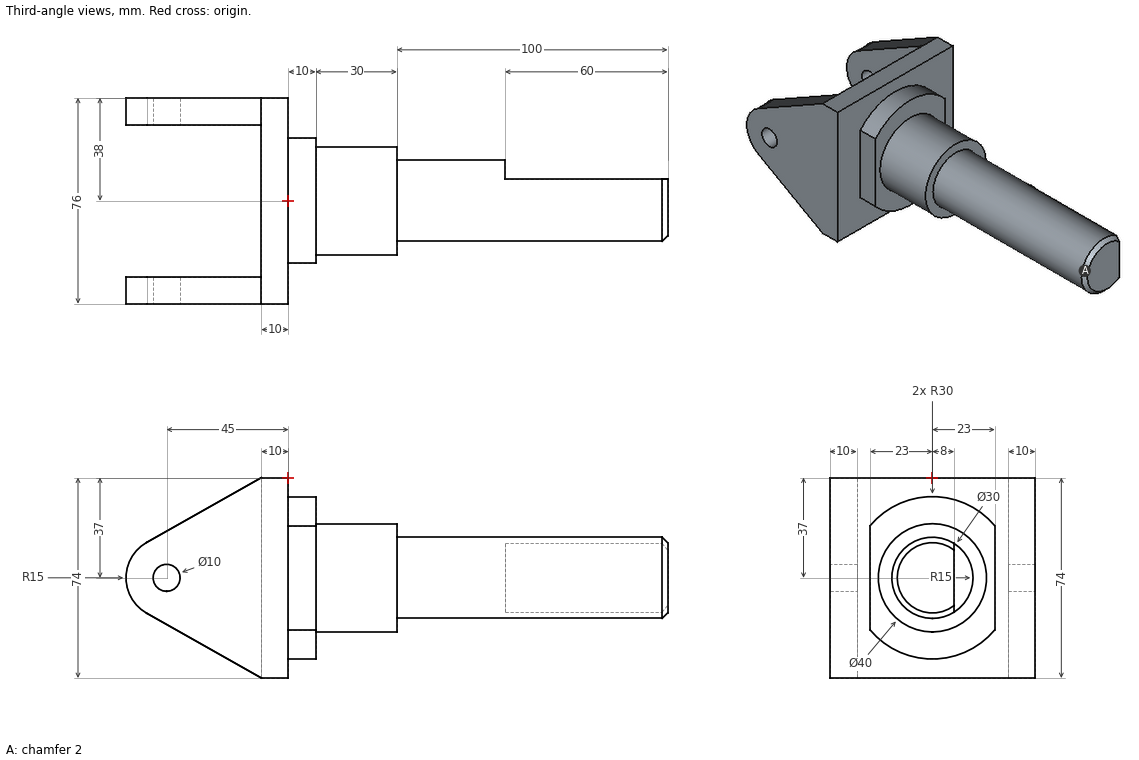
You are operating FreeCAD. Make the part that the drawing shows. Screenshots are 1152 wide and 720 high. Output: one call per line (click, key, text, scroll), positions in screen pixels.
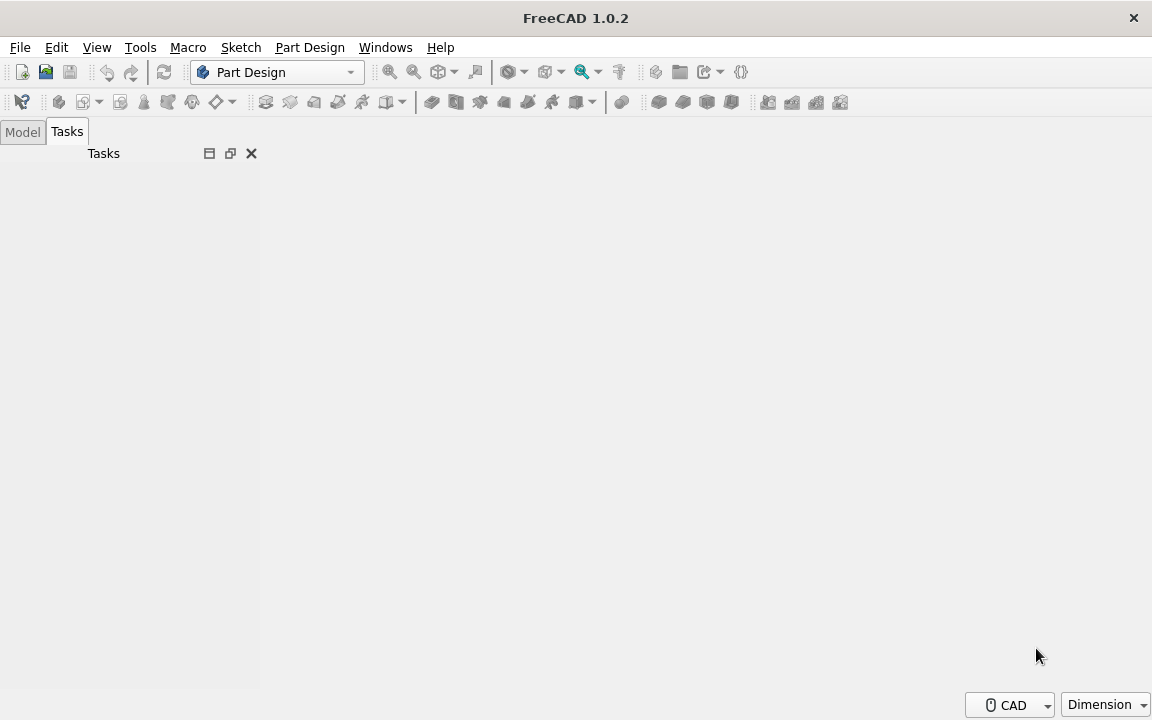
click(22, 72)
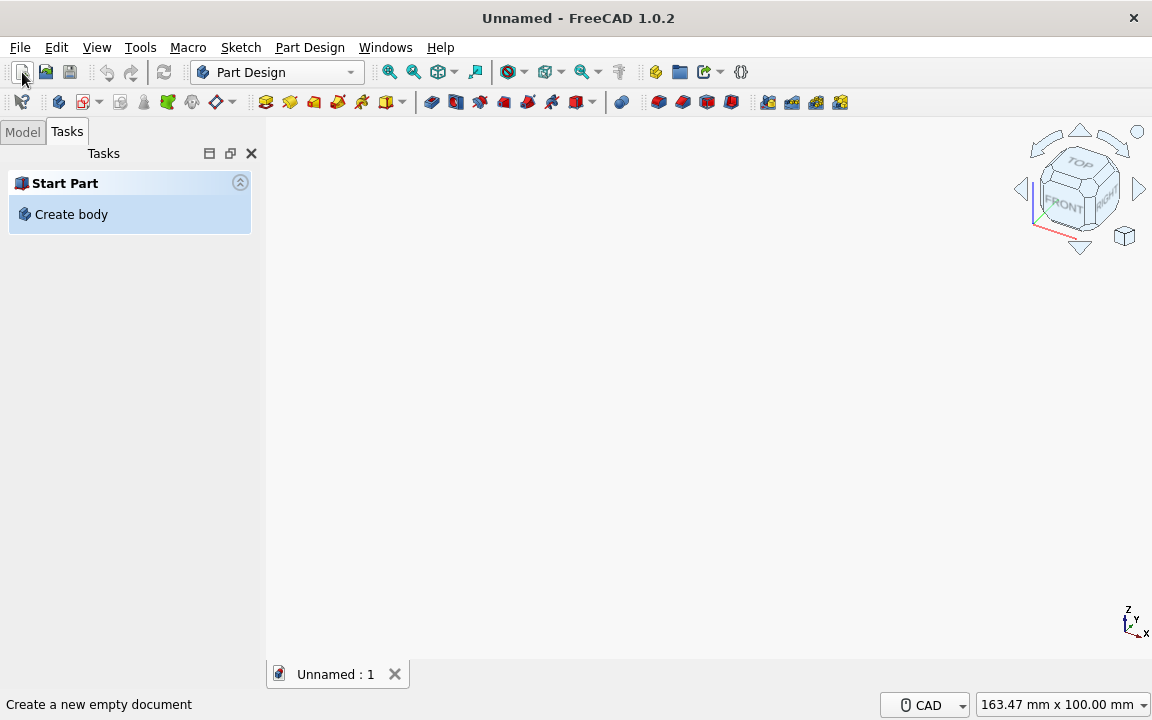
click(84, 102)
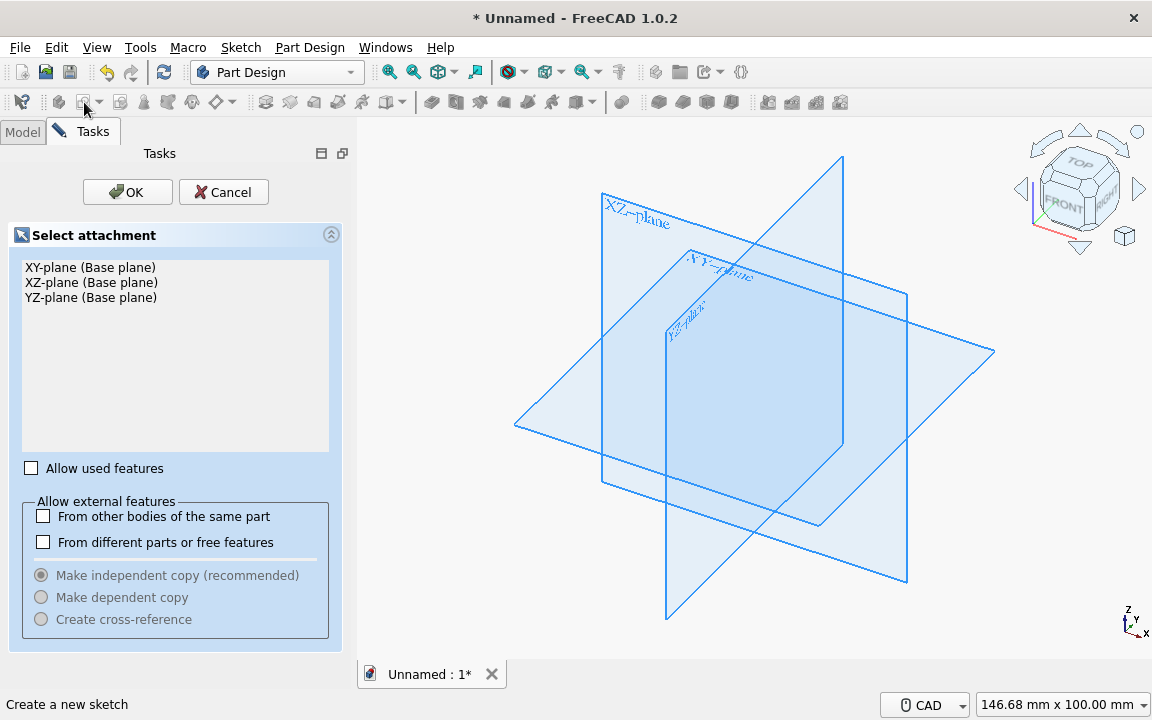
click(82, 268)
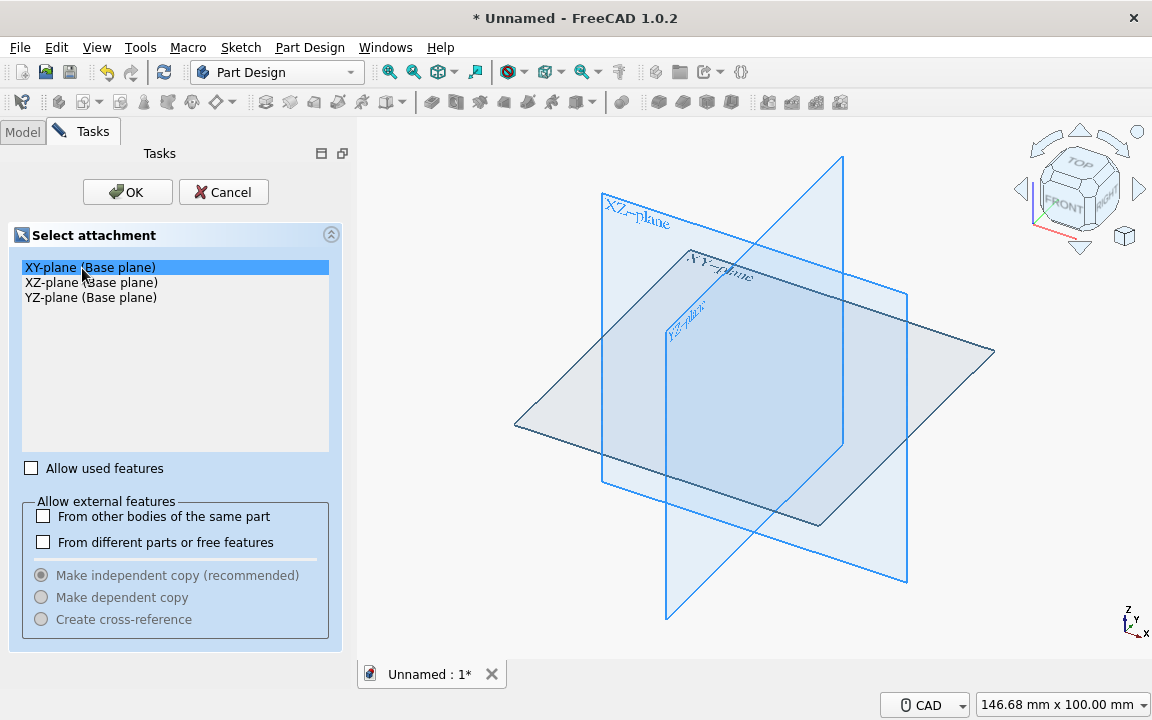
click(128, 192)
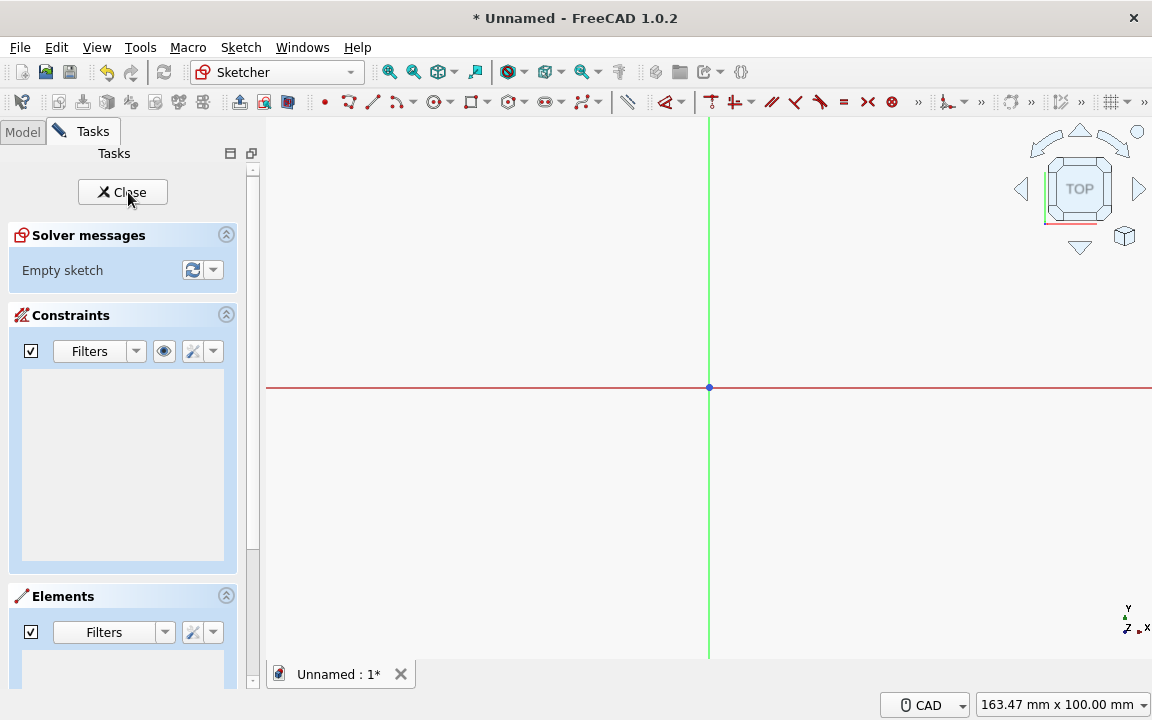
click(472, 102)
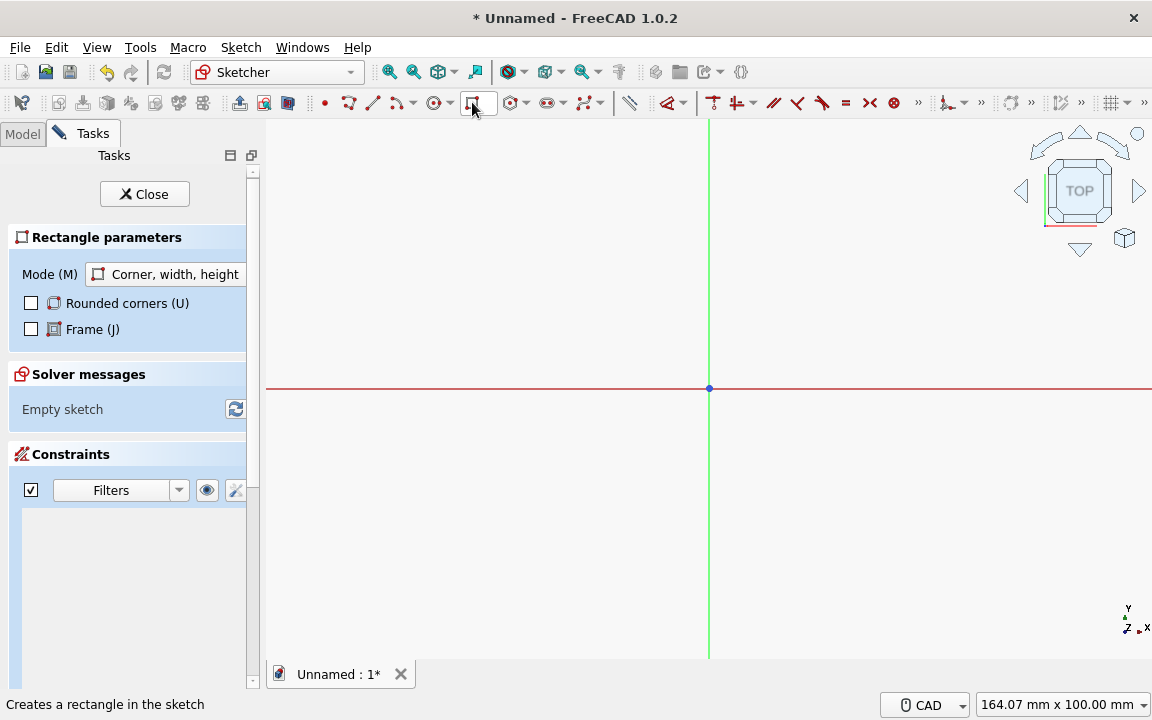
click(655, 184)
click(709, 594)
key(Escape)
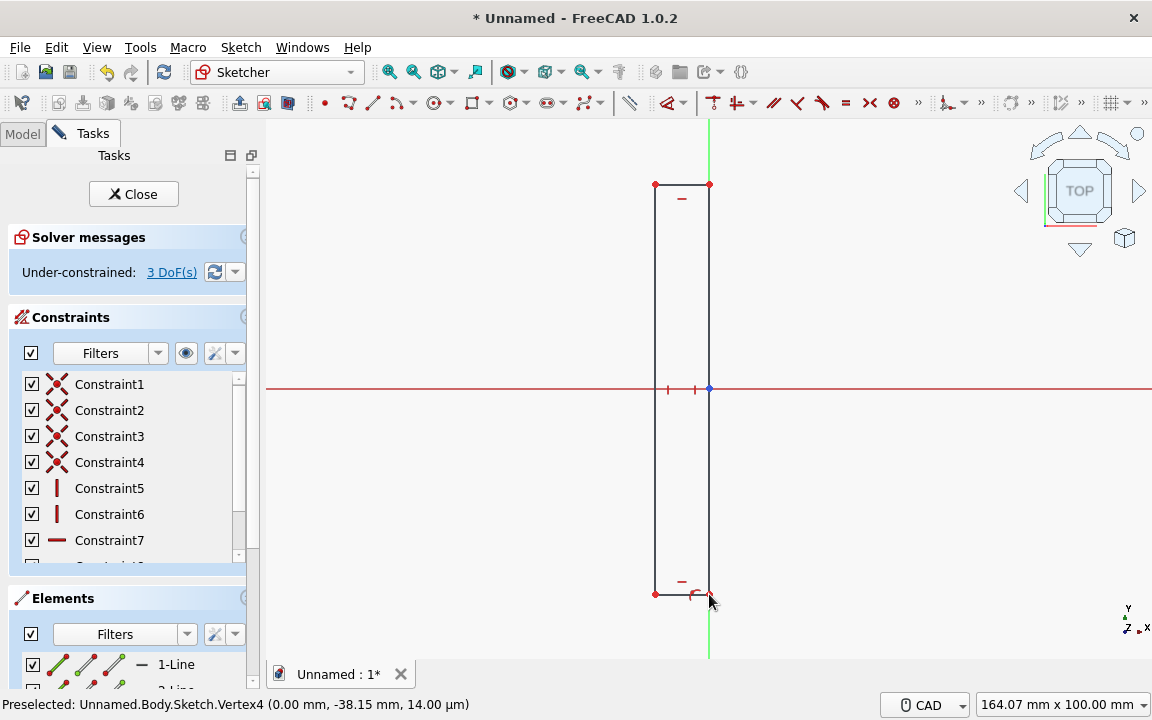
click(668, 104)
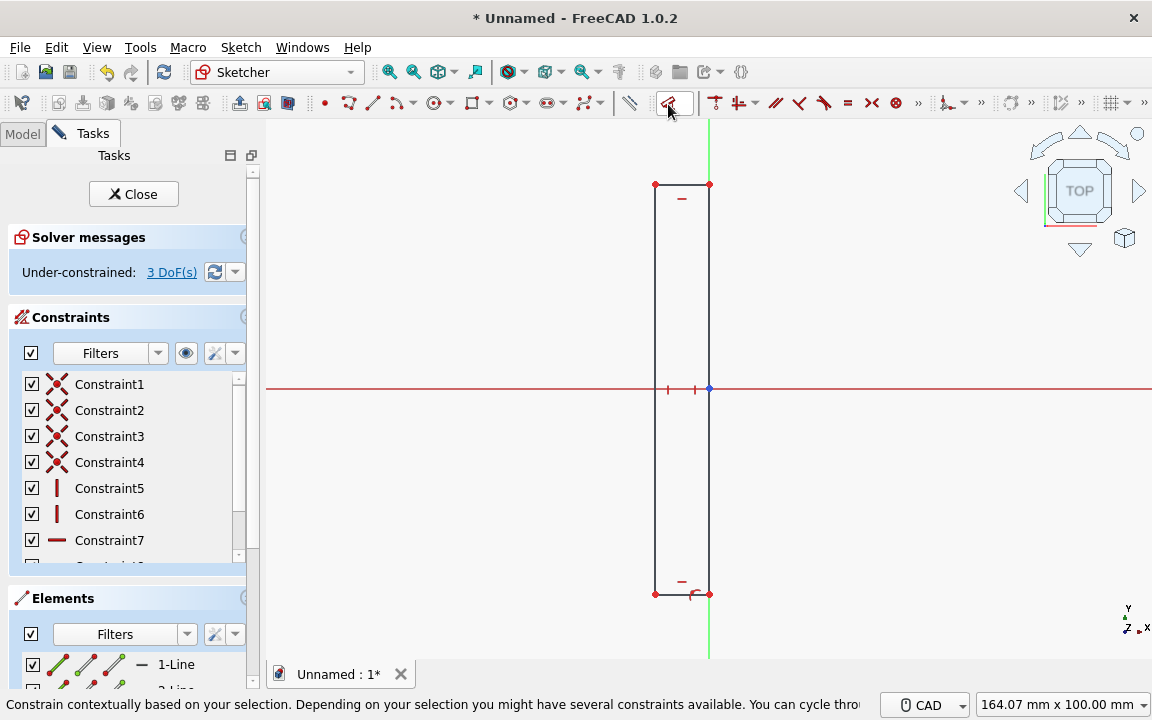
click(655, 308)
click(621, 296)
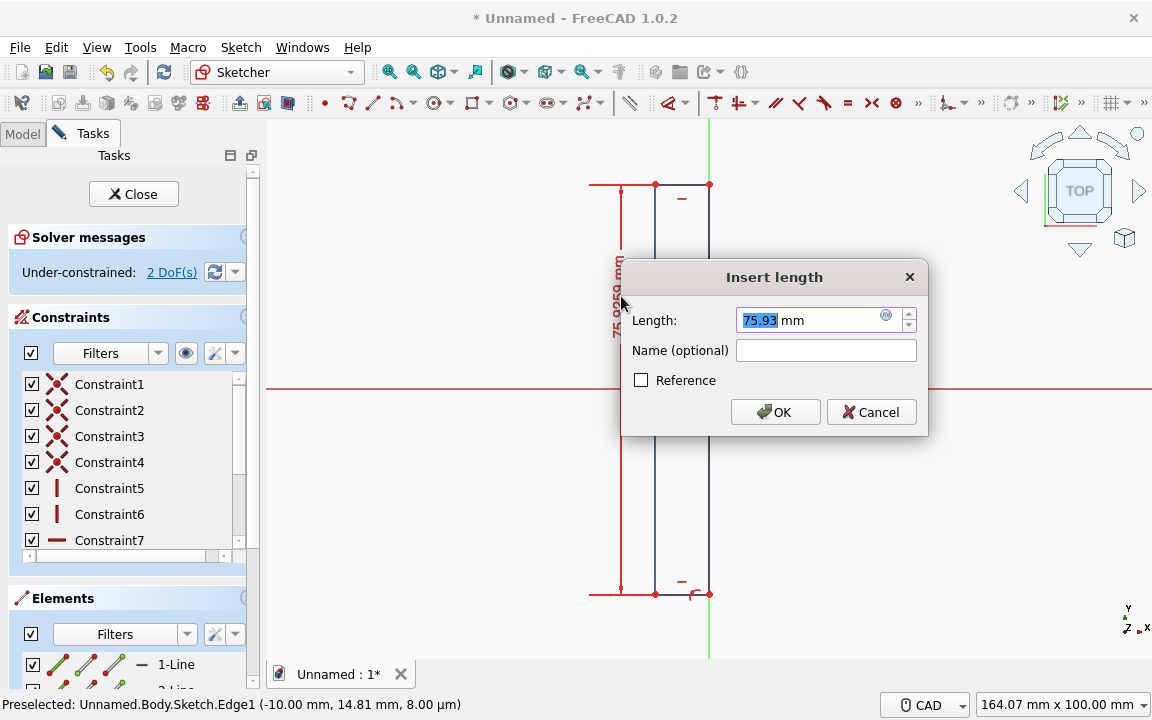
text(76)
key(Return)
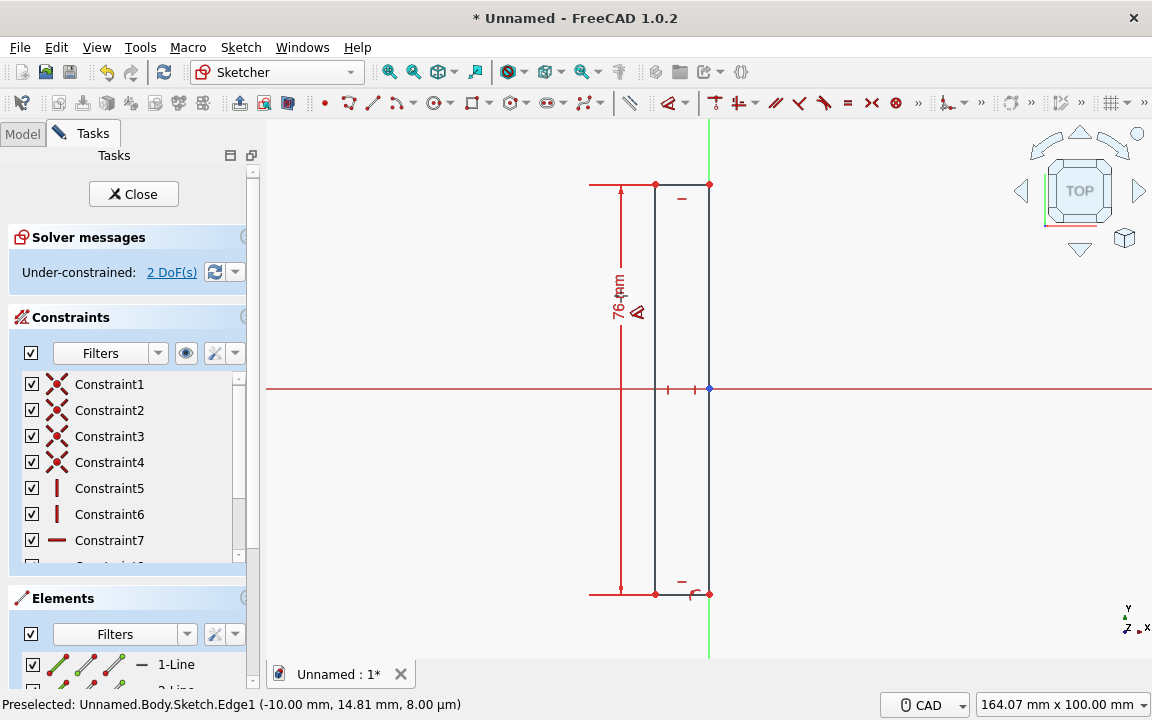
click(671, 595)
click(682, 629)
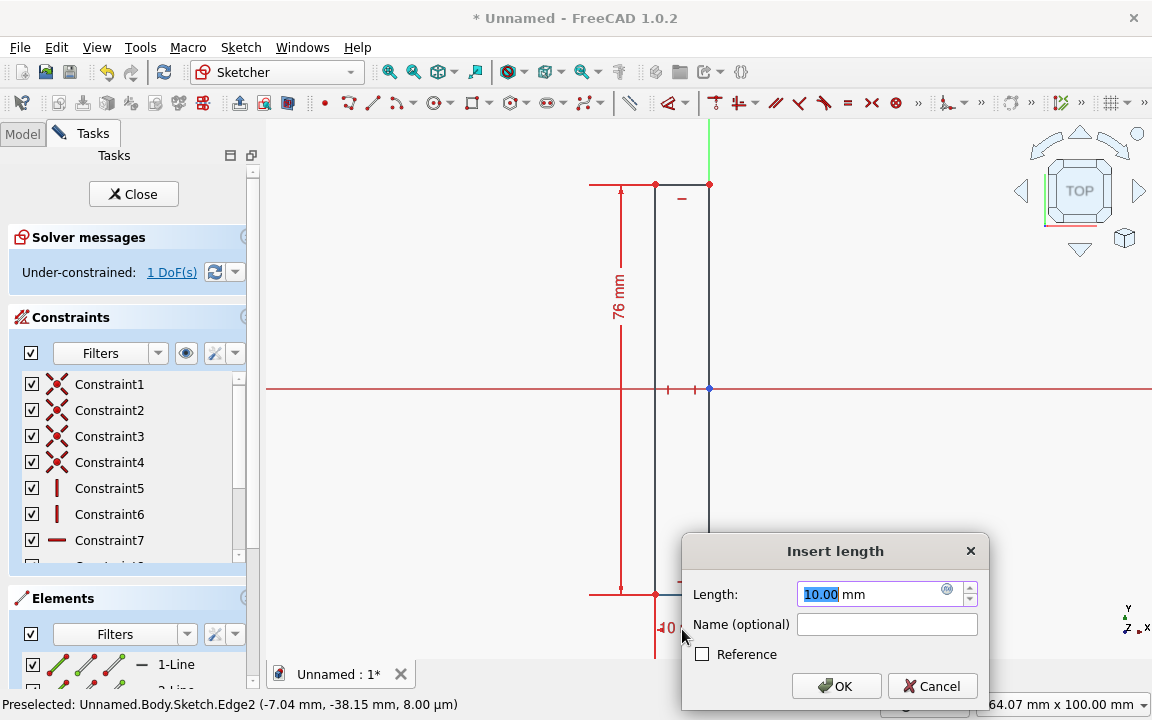
text(10)
key(Return)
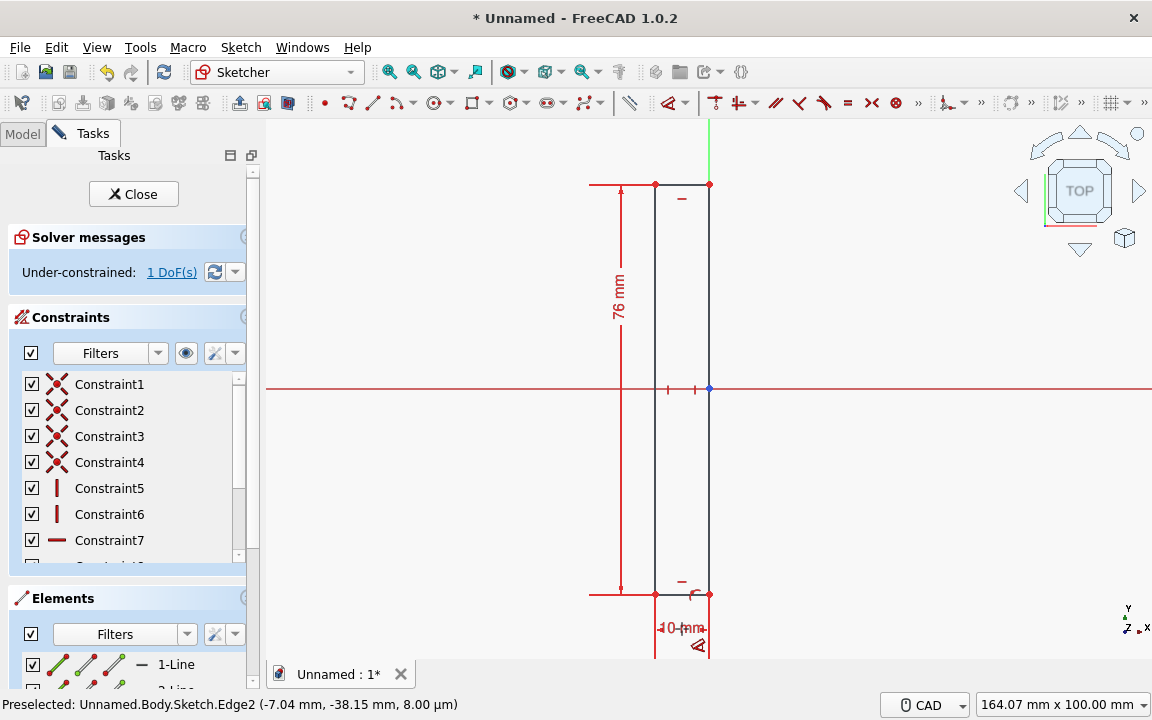
click(655, 185)
click(743, 287)